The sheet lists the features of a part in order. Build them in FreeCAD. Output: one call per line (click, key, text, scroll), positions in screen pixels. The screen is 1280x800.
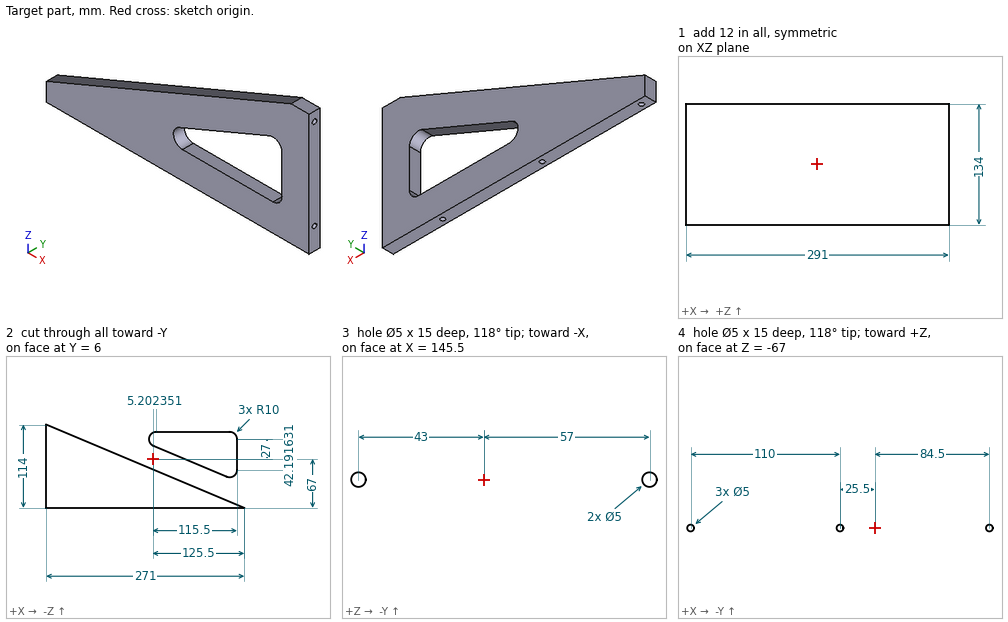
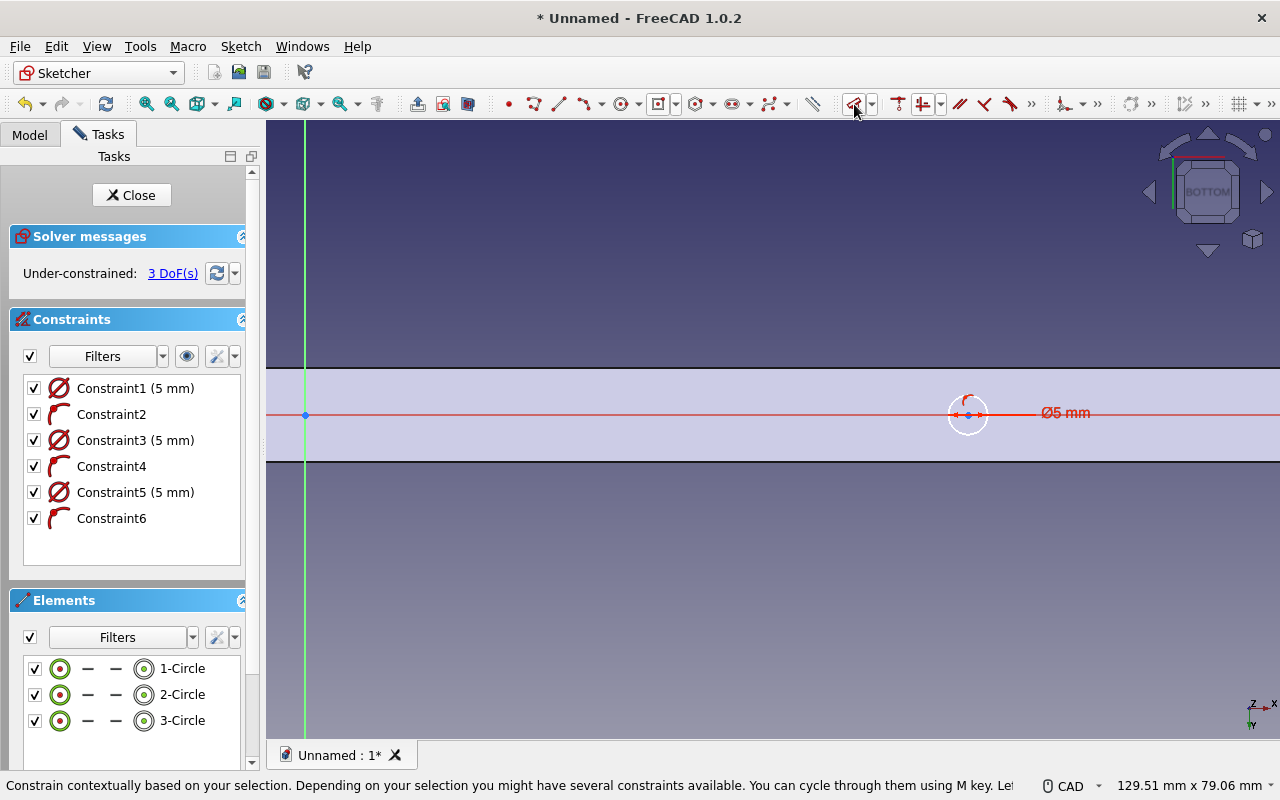
scroll(963, 436, down, 6)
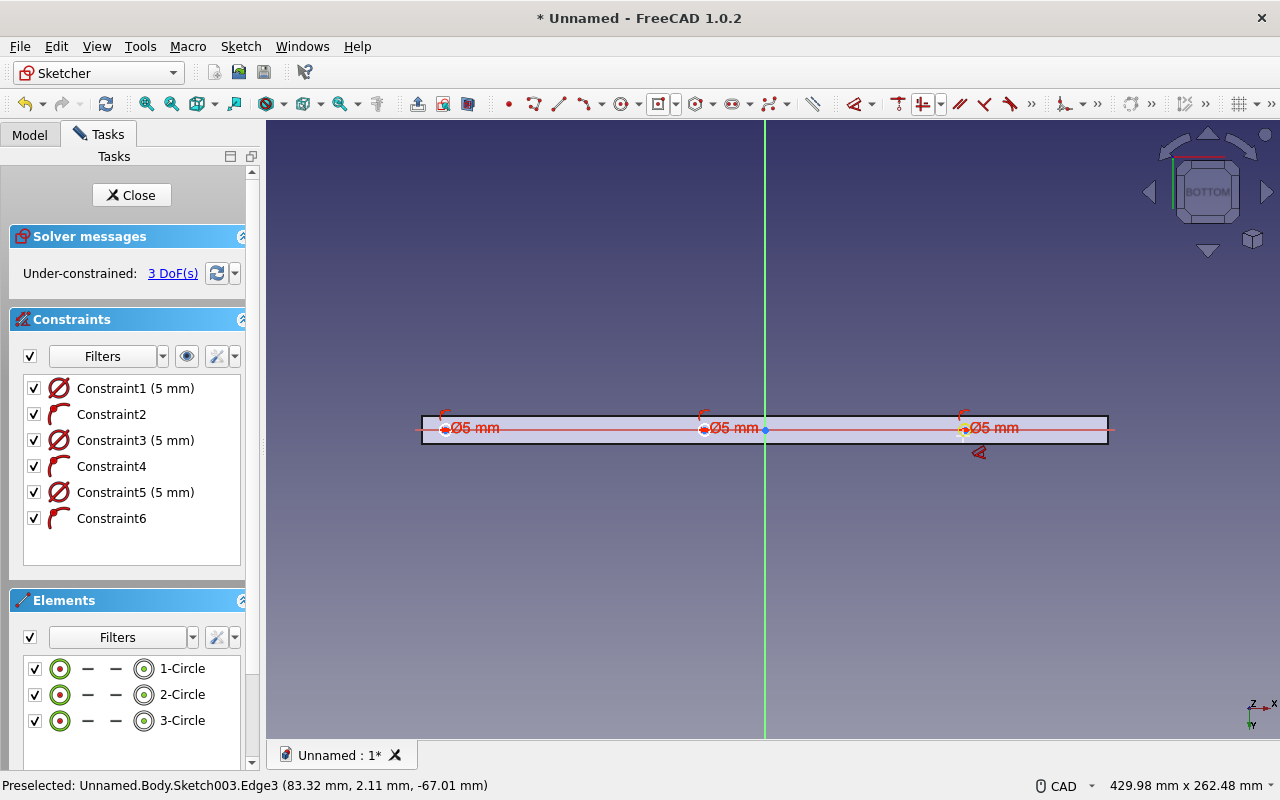
click(705, 430)
click(735, 464)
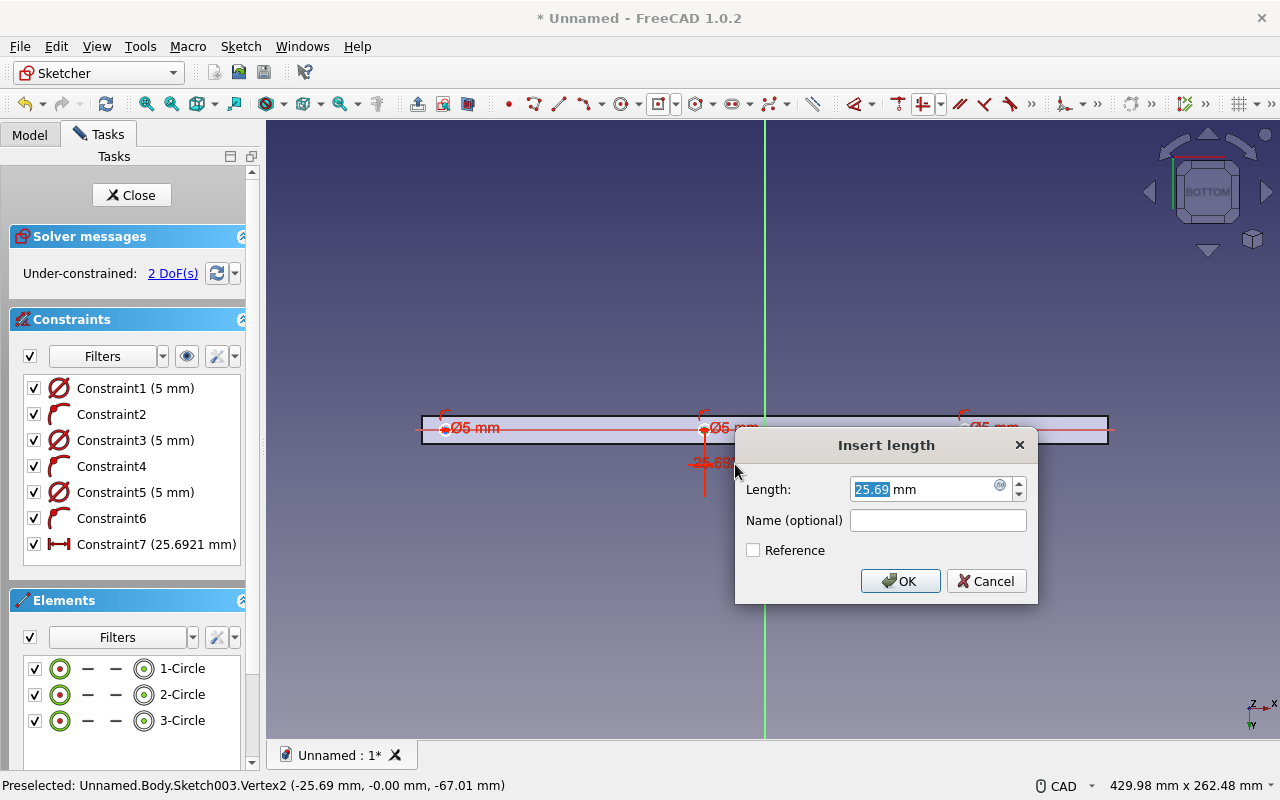
text(25.5)
key(Return)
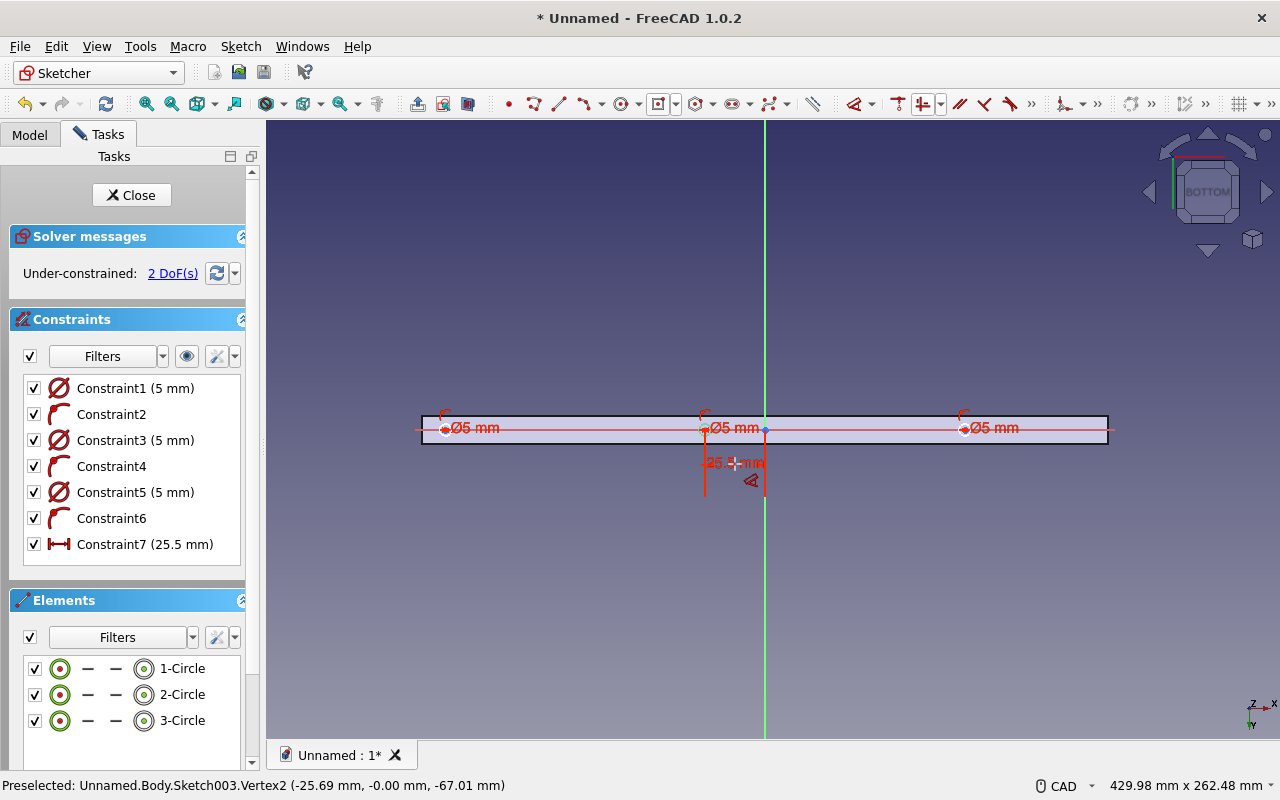
click(965, 430)
click(865, 464)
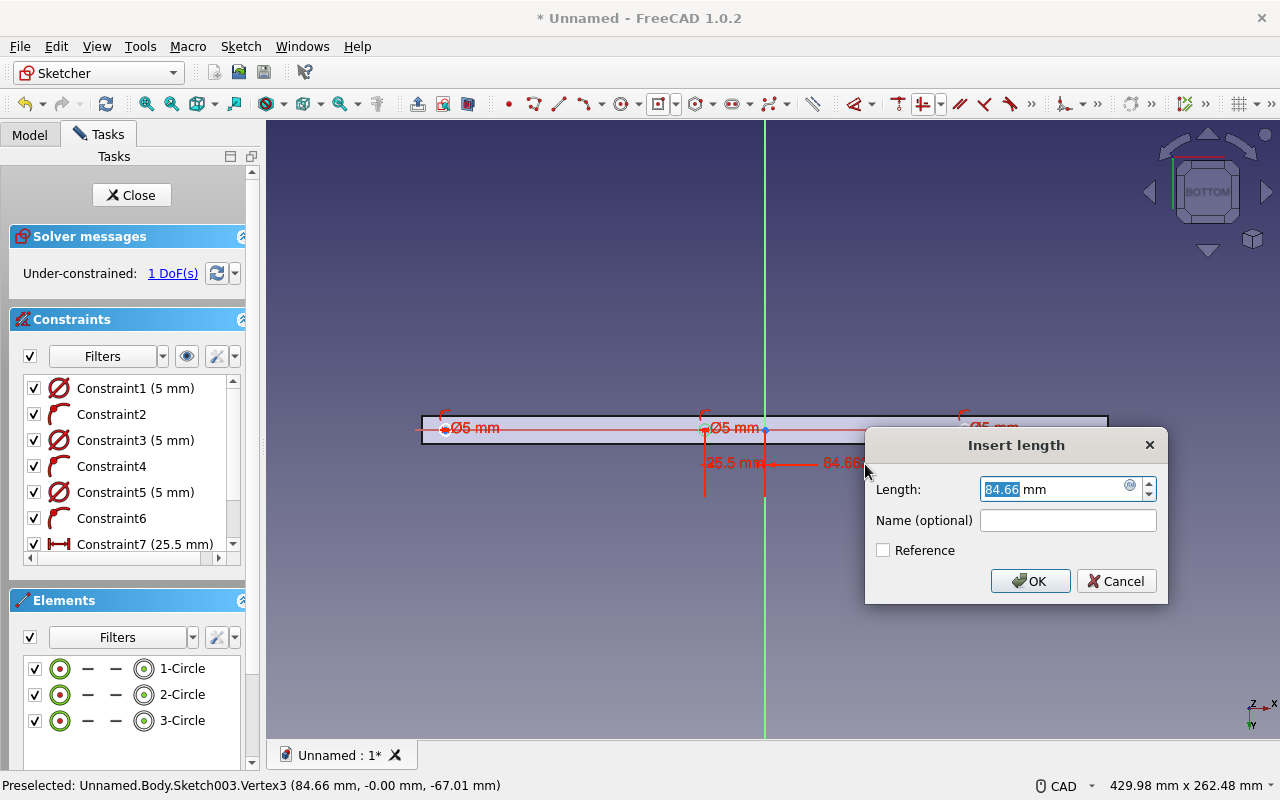
text(84.5)
key(Return)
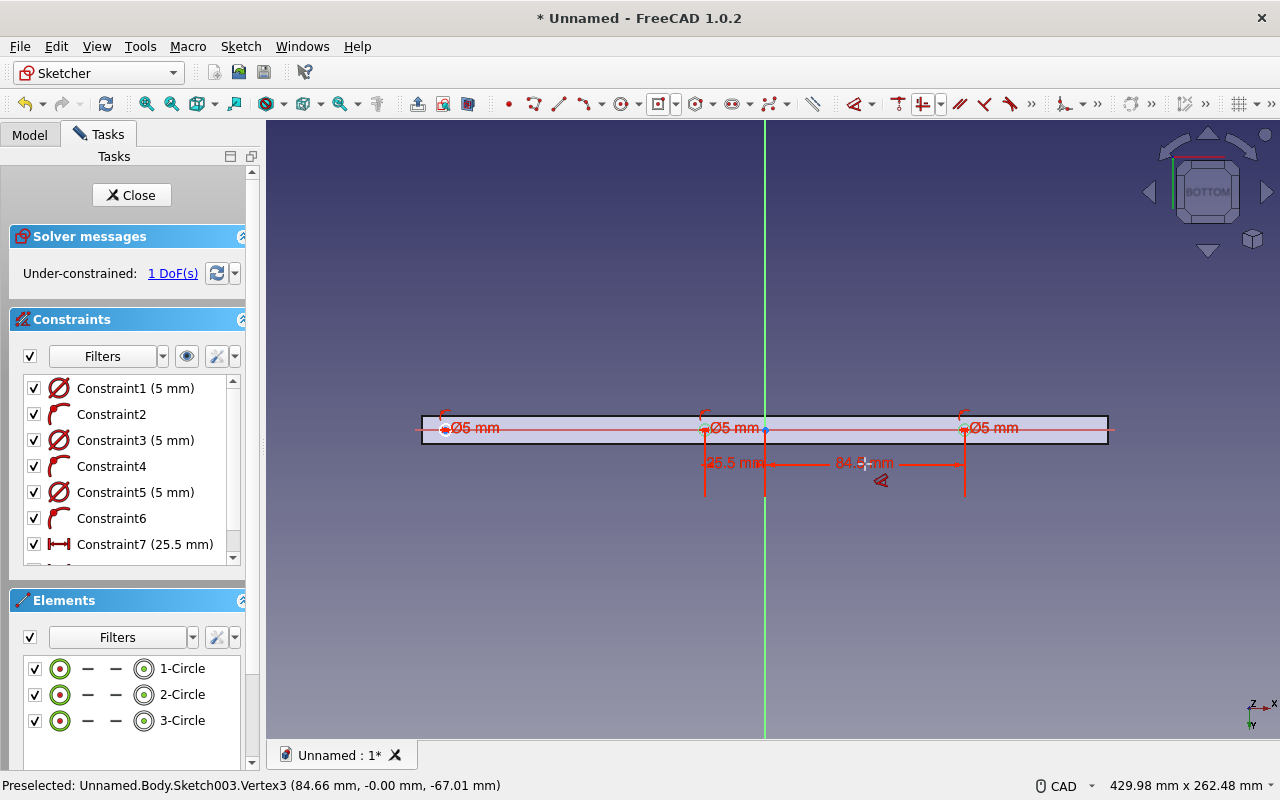
click(446, 430)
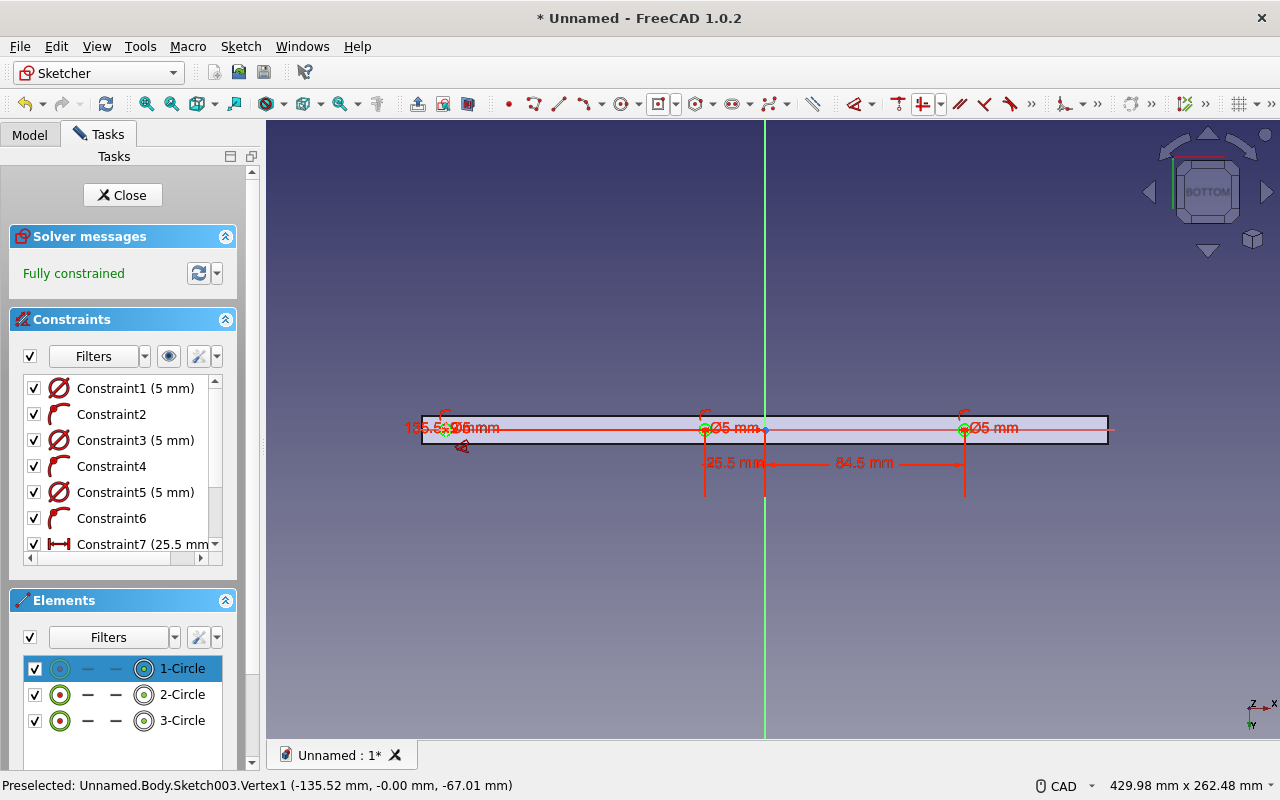
click(705, 430)
click(575, 464)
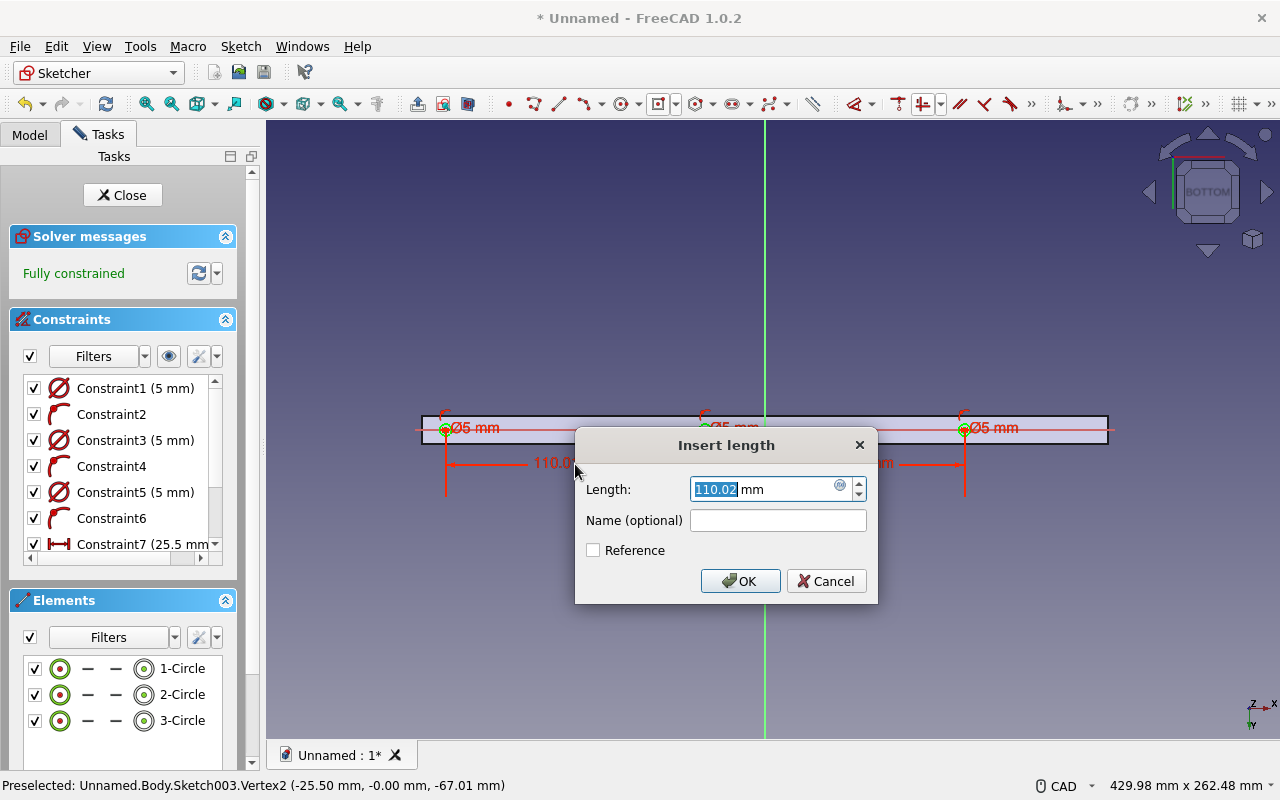
text(110)
key(Return)
key(Escape)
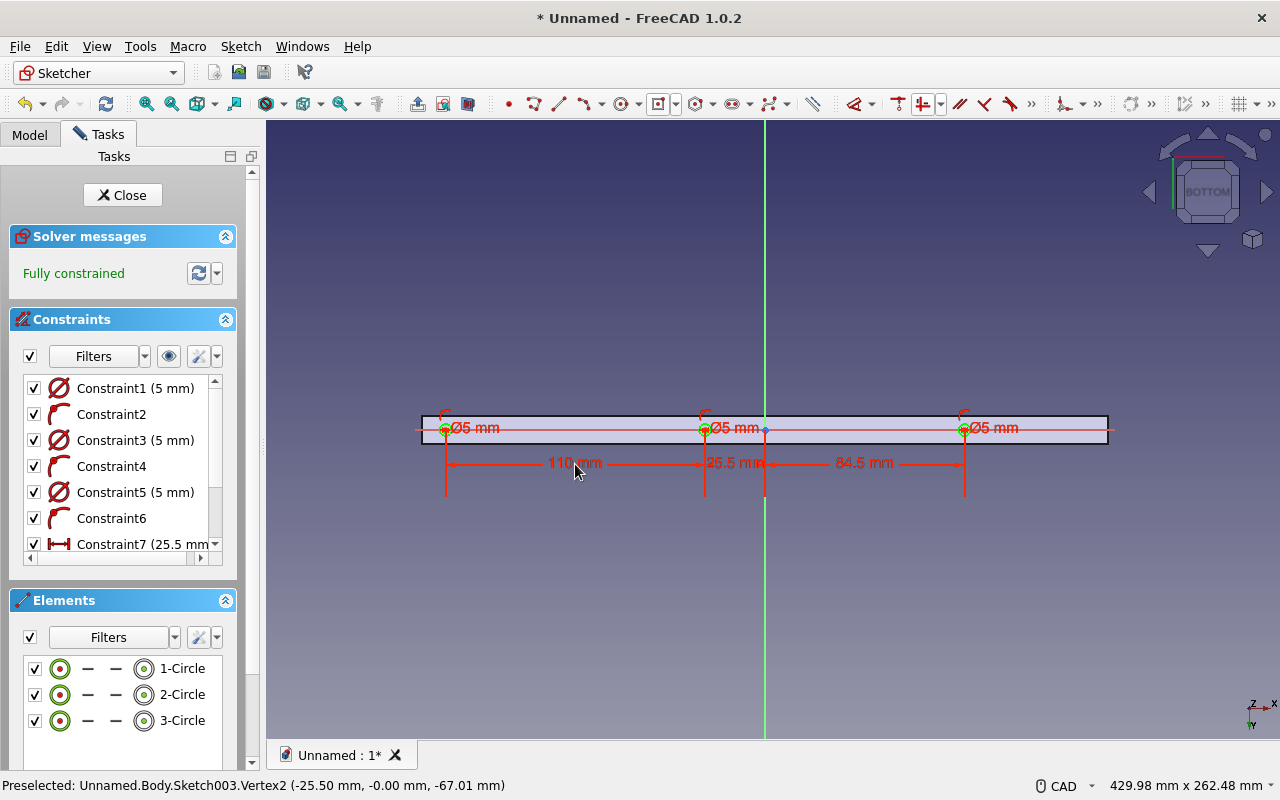
click(123, 195)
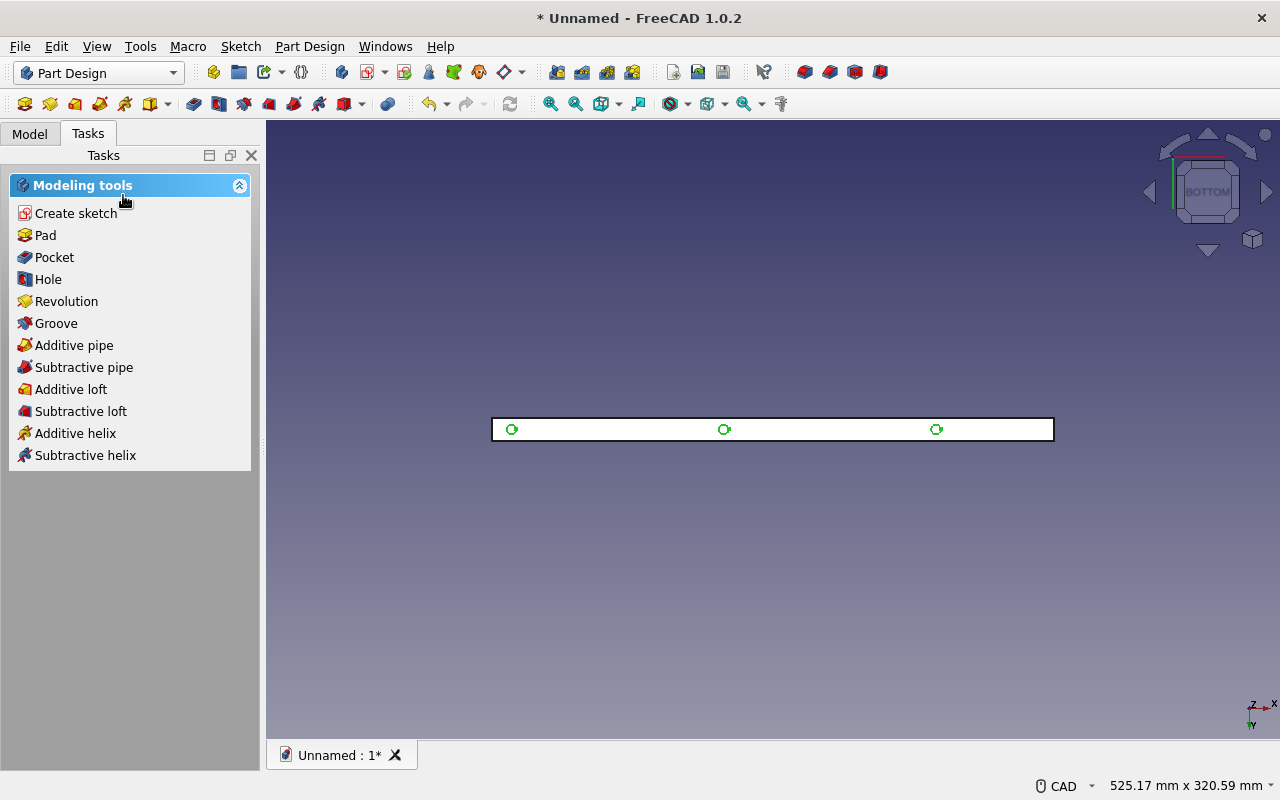
click(219, 104)